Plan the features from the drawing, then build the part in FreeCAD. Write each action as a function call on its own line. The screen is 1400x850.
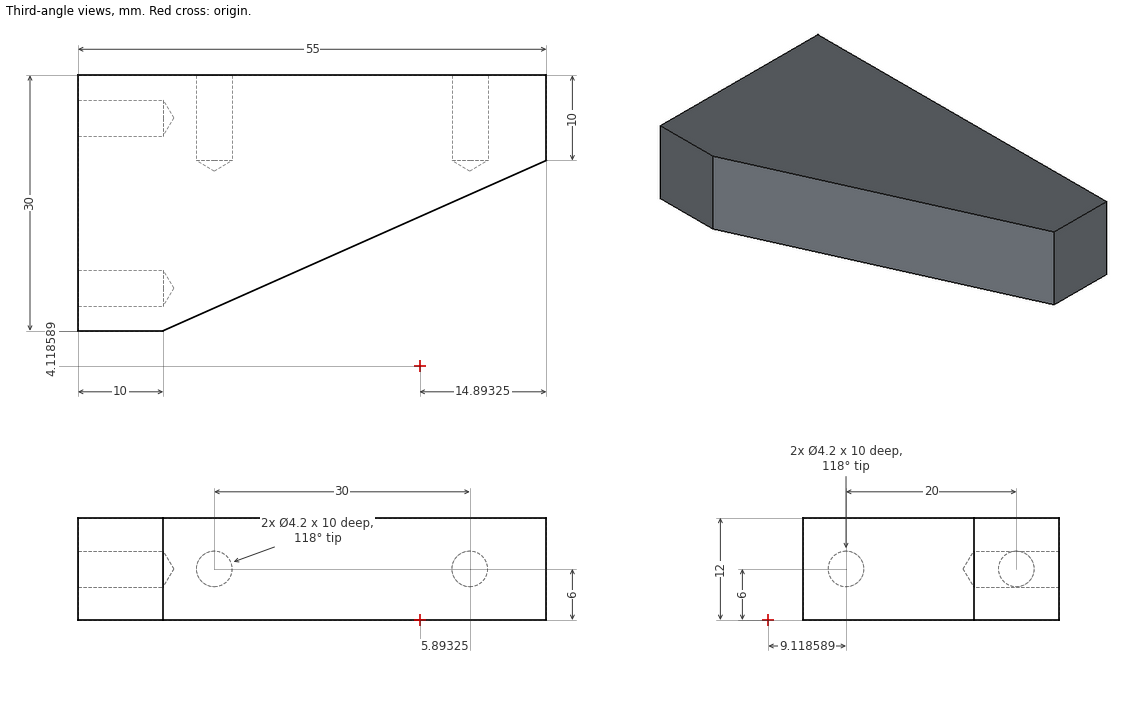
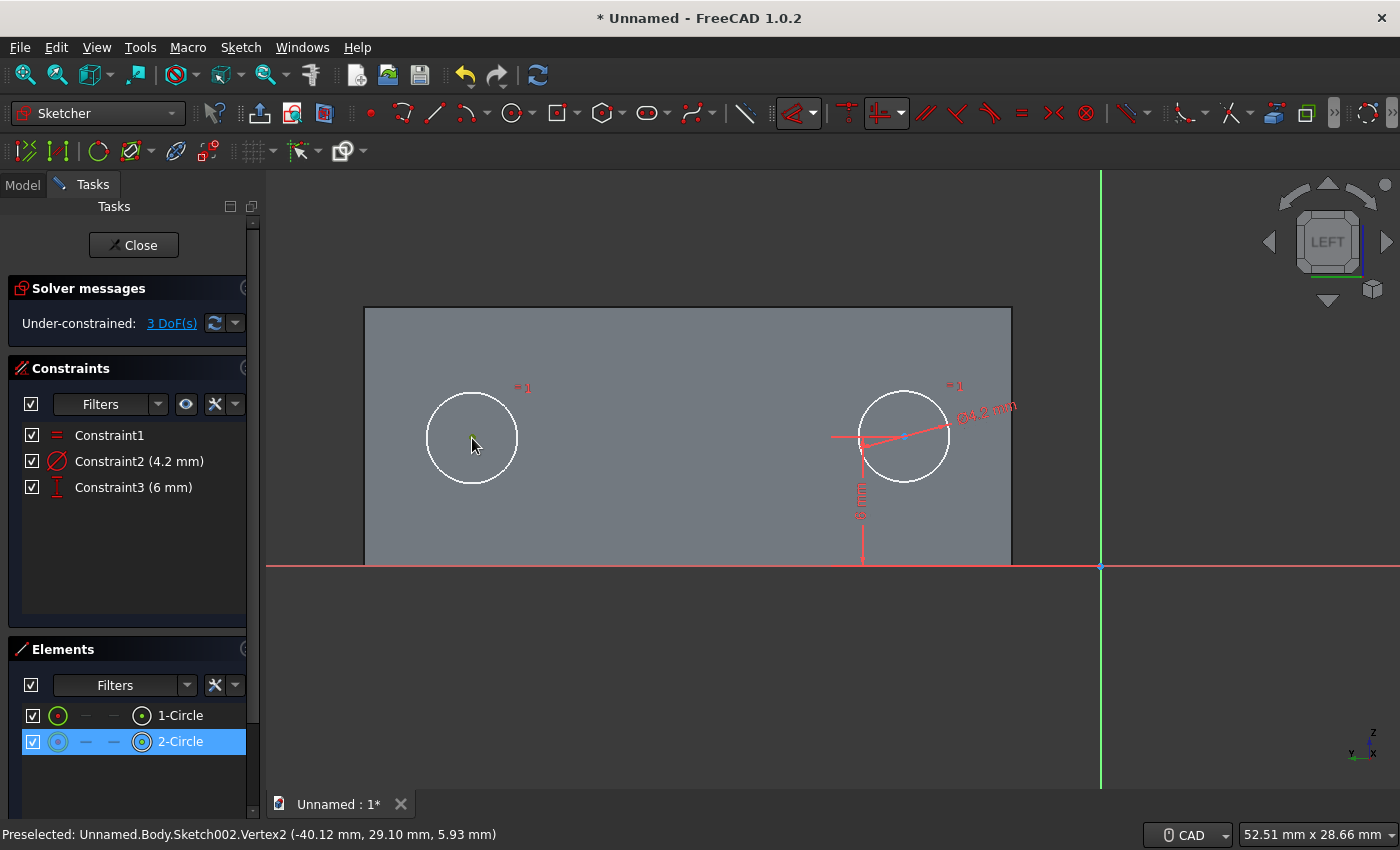
key(i)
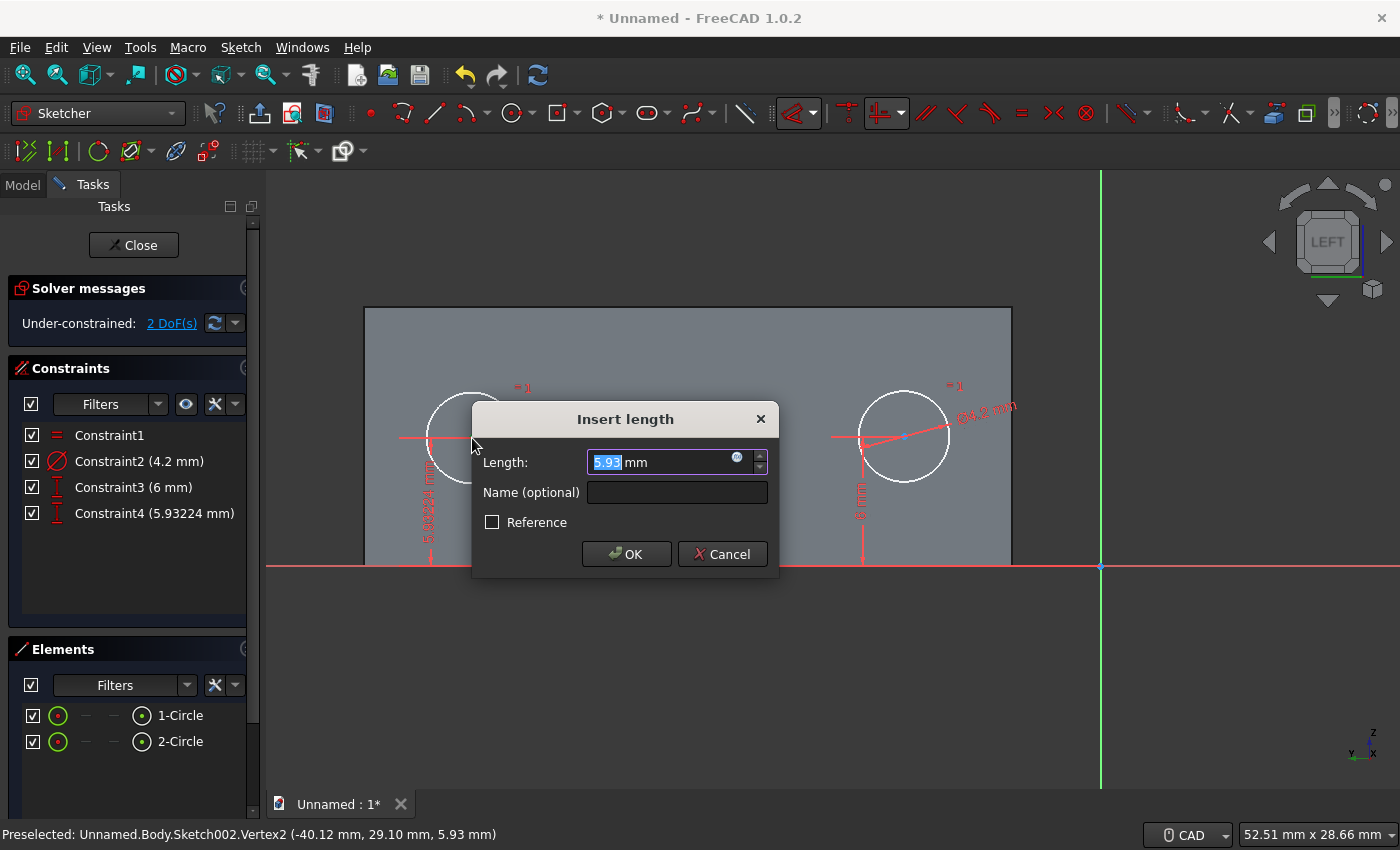
text(6)
key(Return)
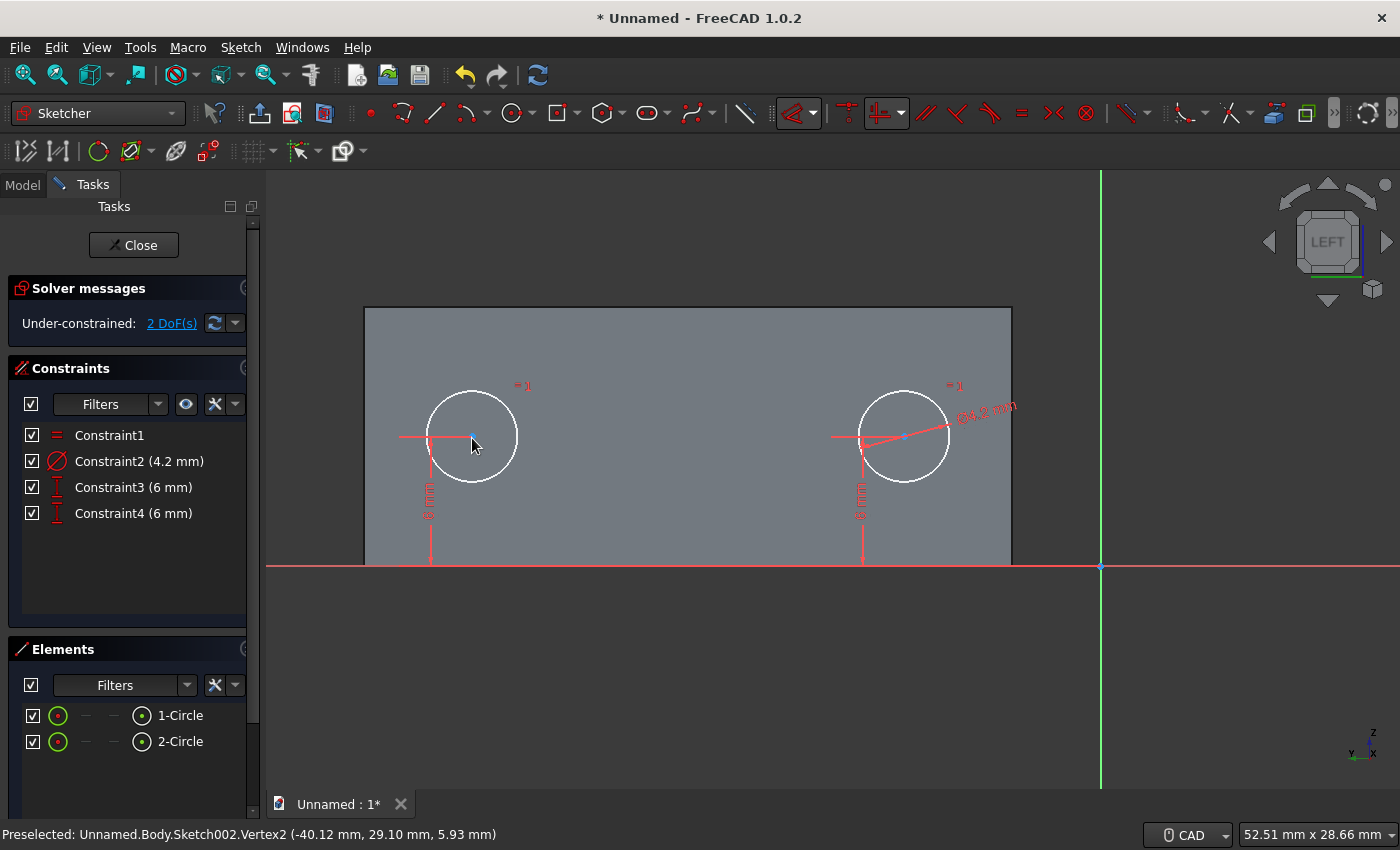
click(904, 437)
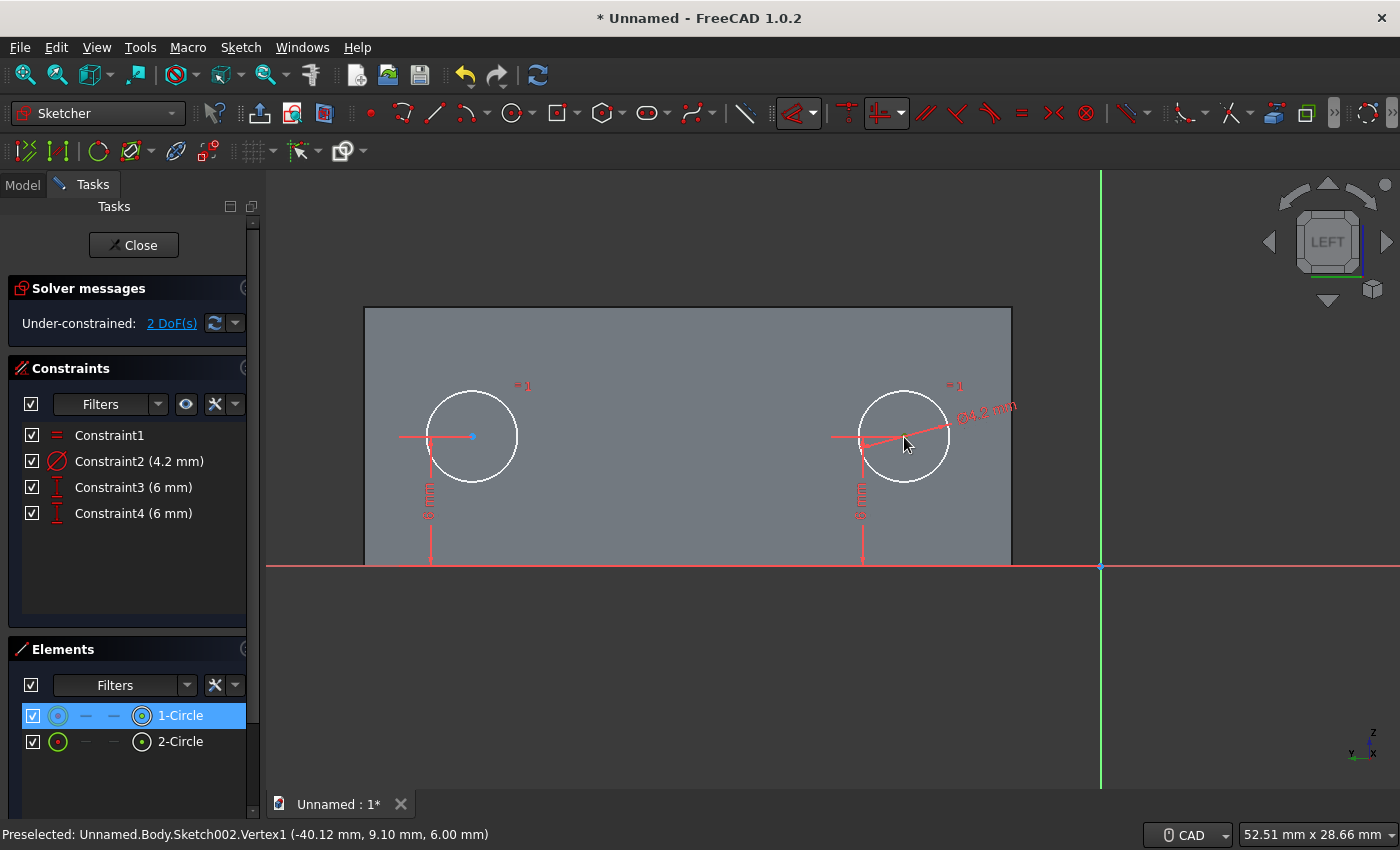
click(472, 437)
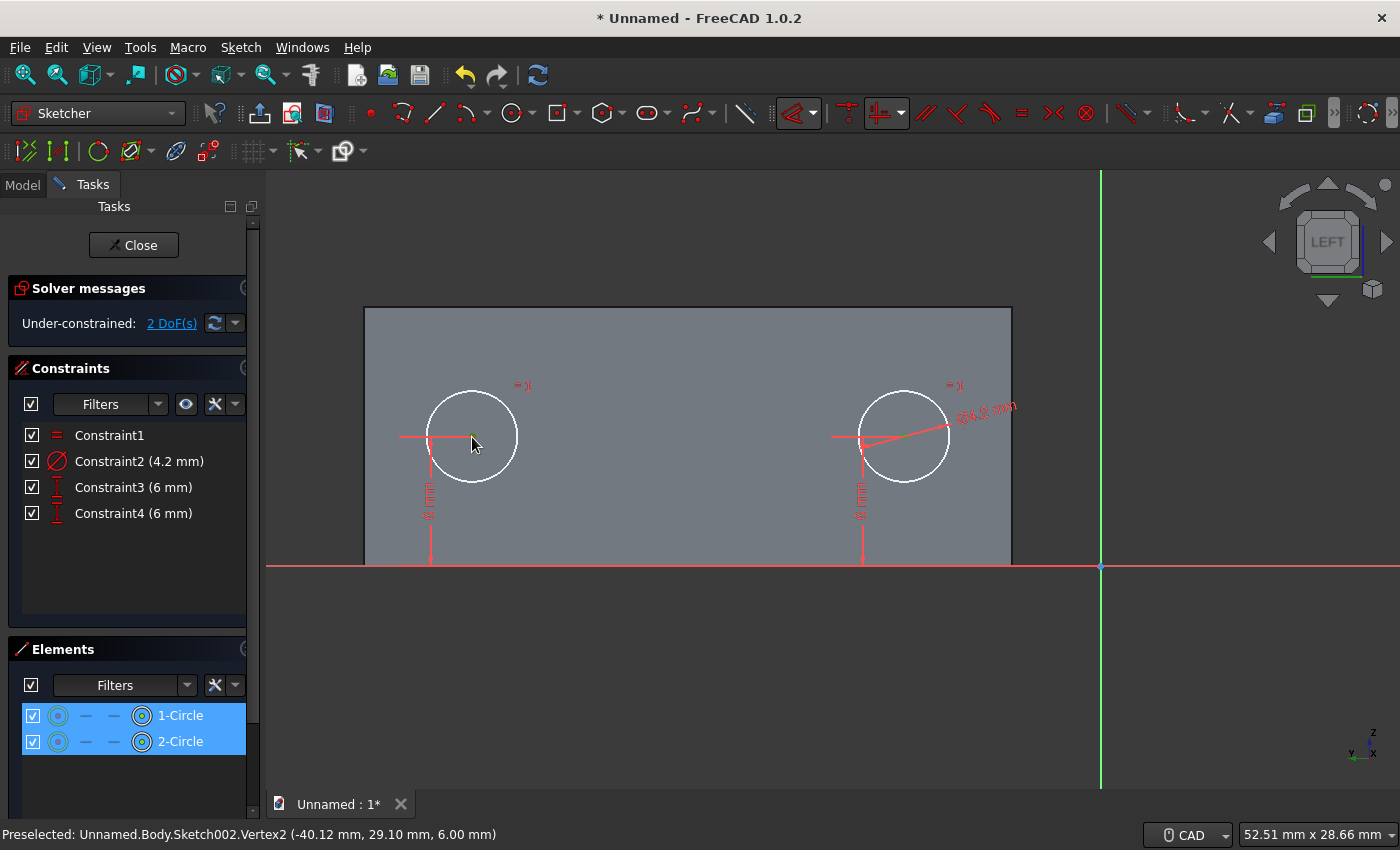
click(816, 114)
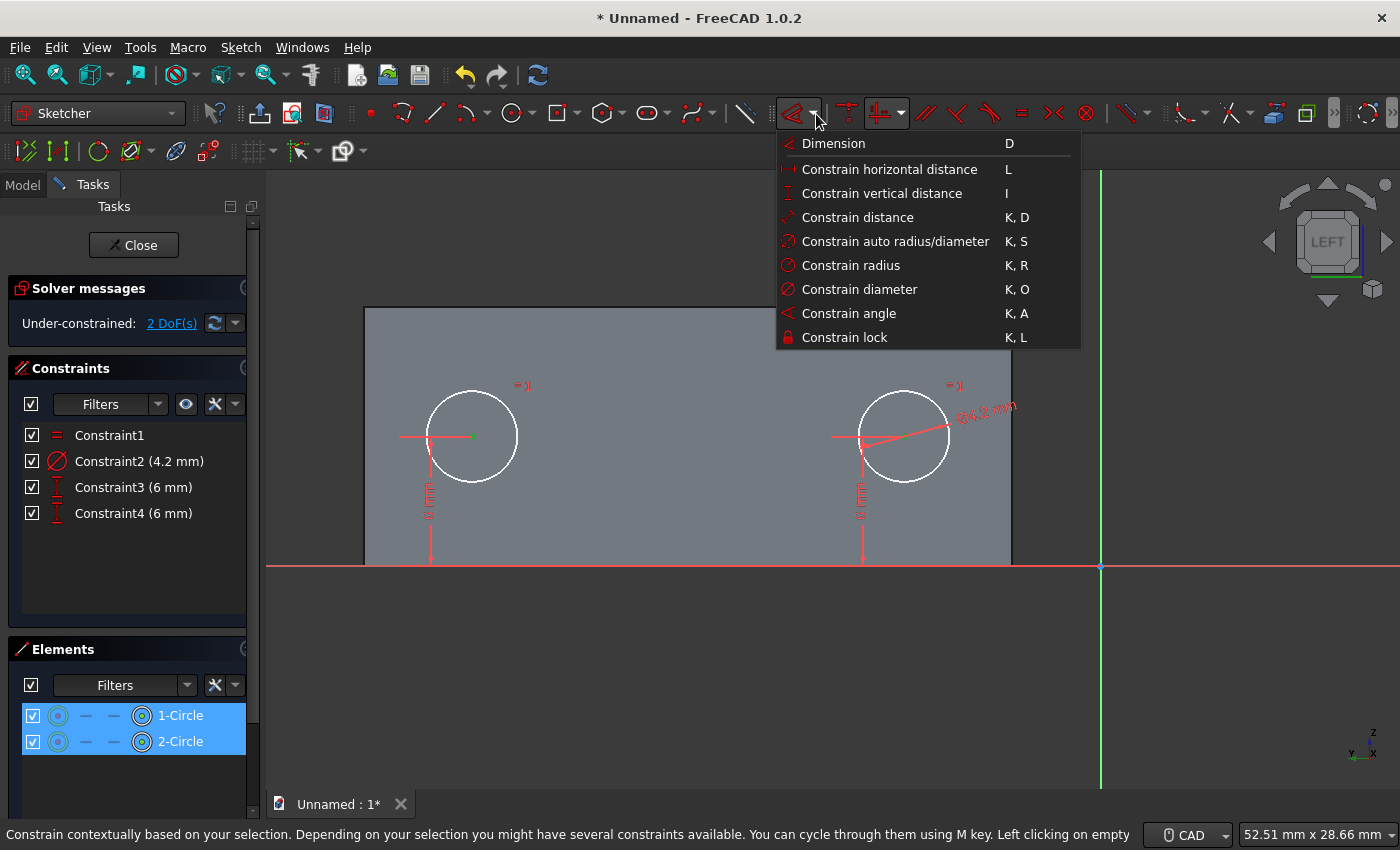
click(929, 169)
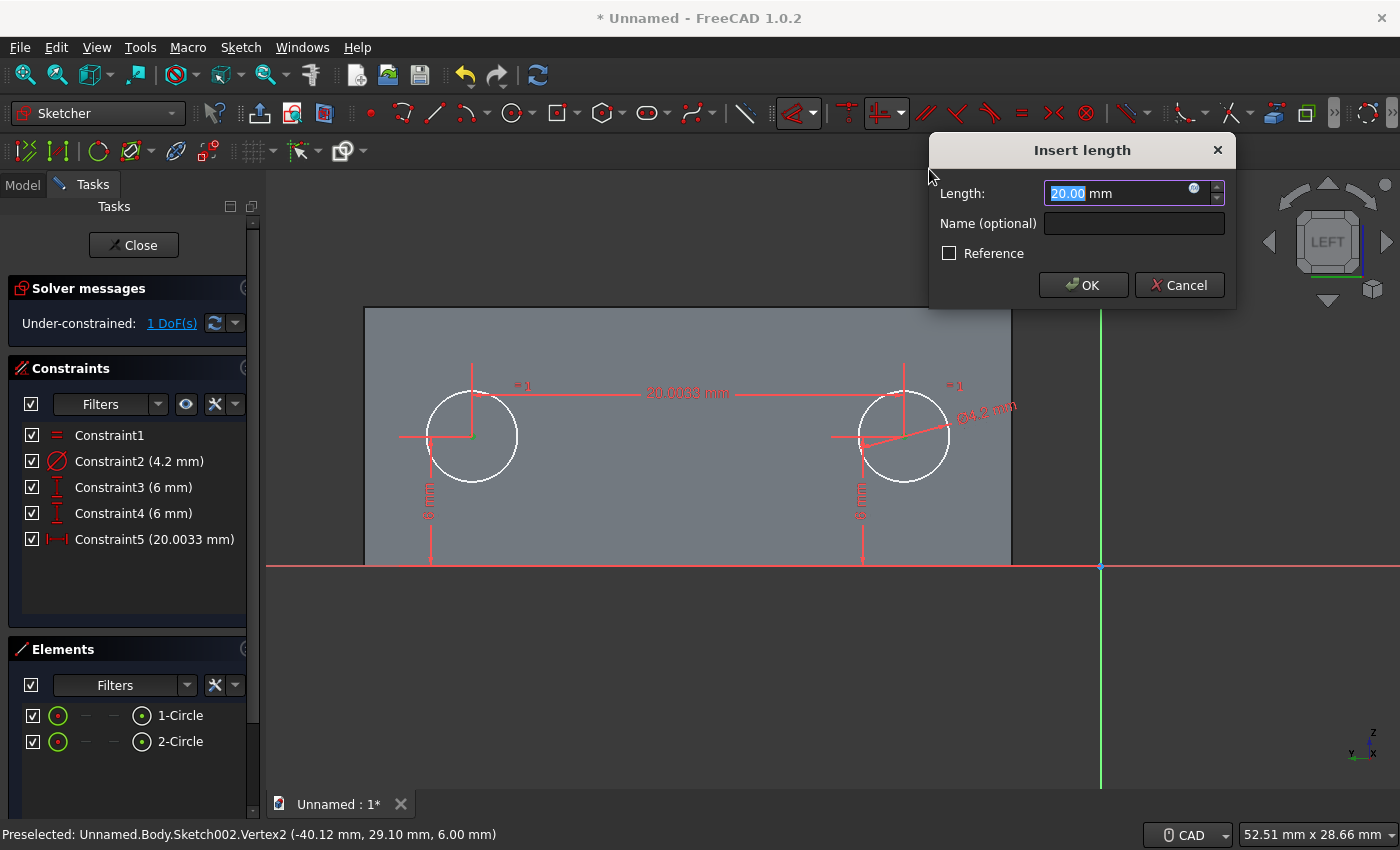
text(20)
key(Return)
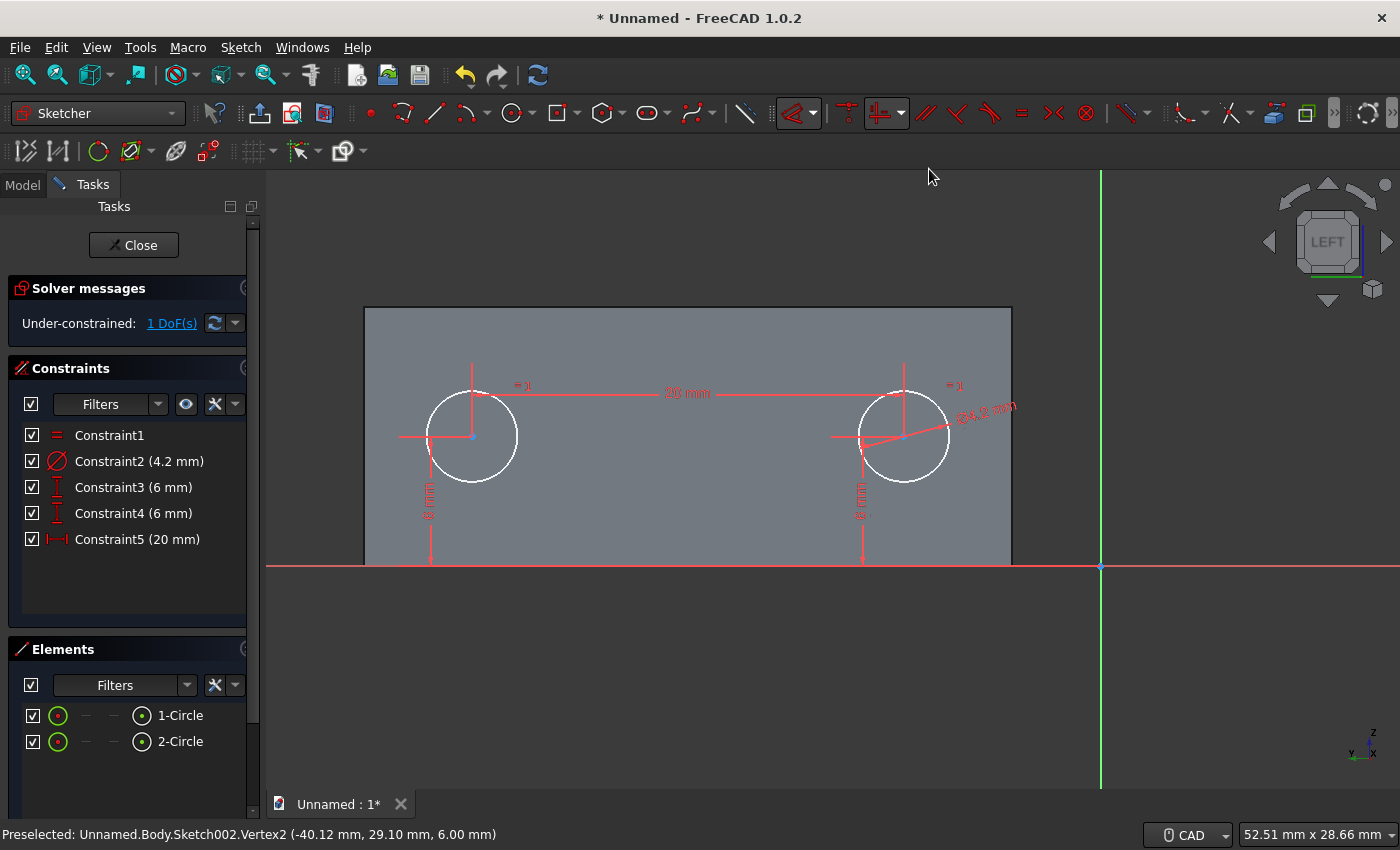
click(904, 437)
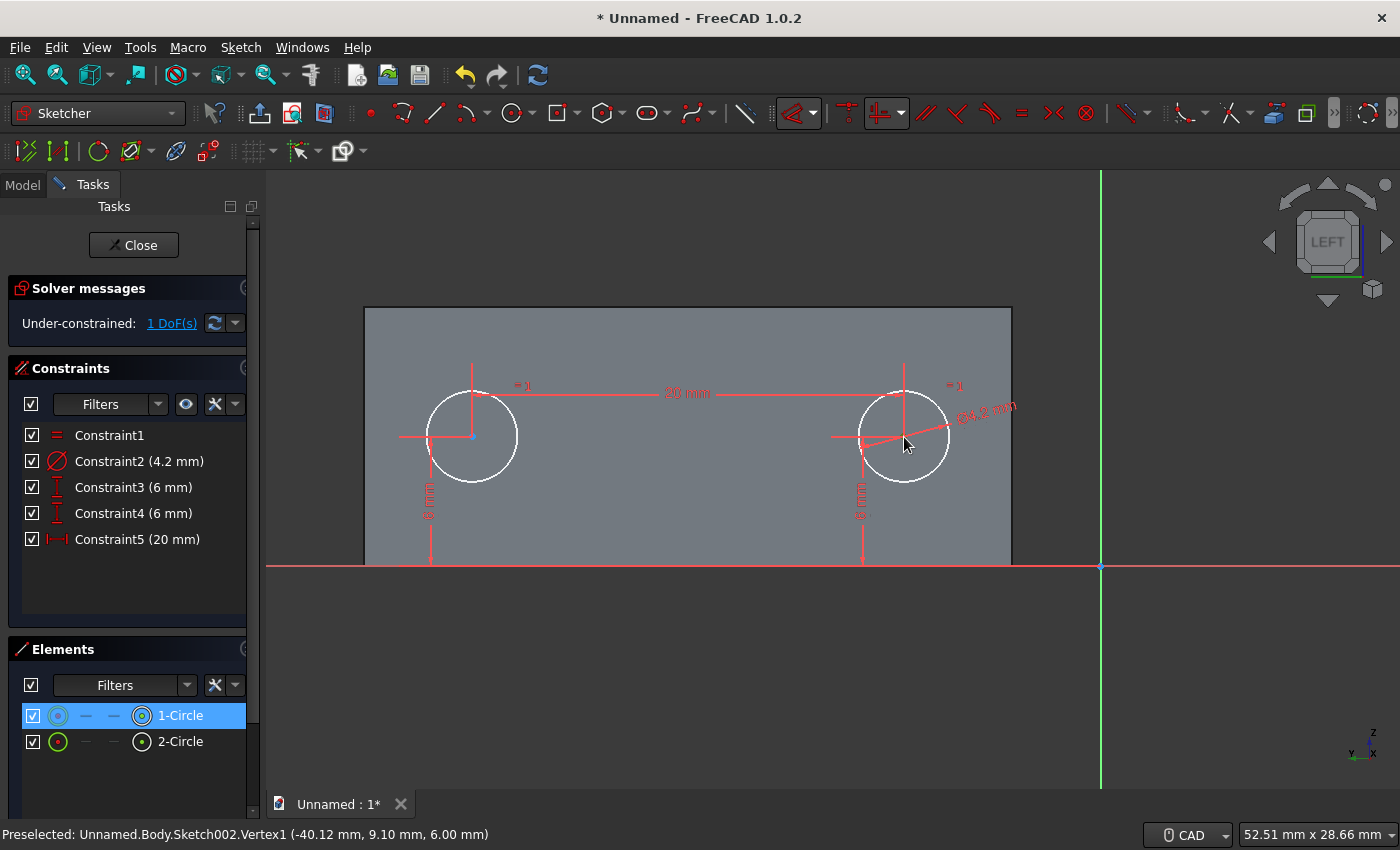
key(l)